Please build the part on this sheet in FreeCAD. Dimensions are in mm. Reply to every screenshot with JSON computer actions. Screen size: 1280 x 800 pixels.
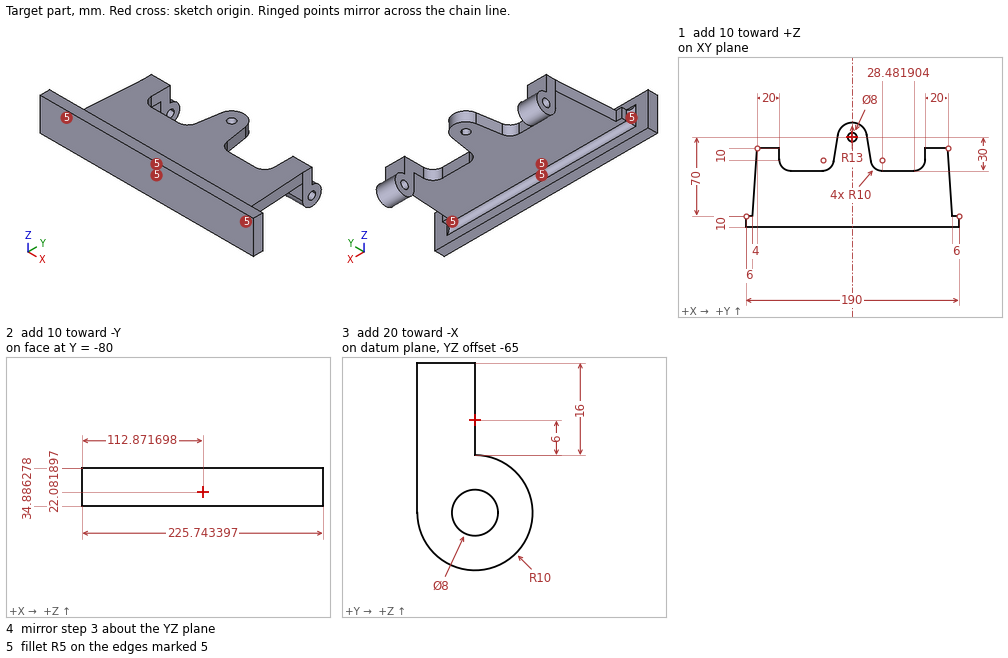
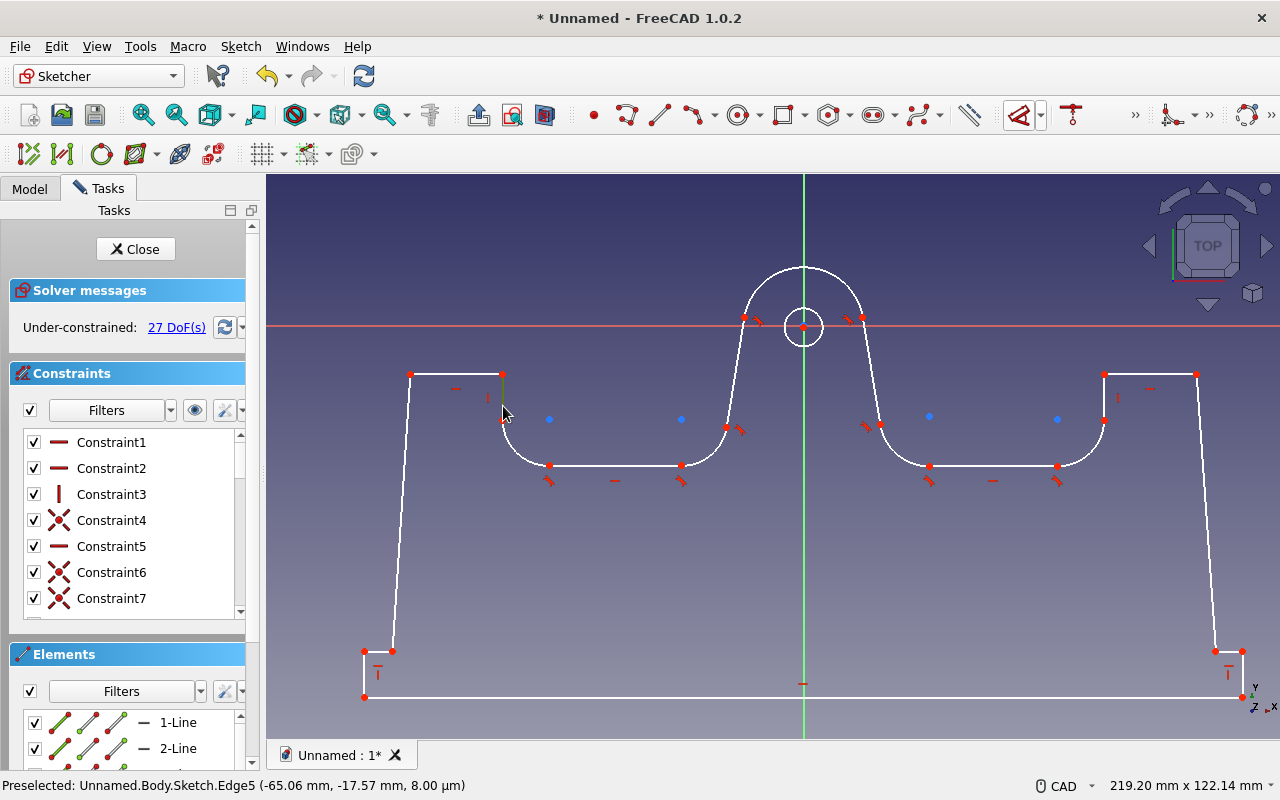
{"action": "left_click", "coordinate": [508, 441]}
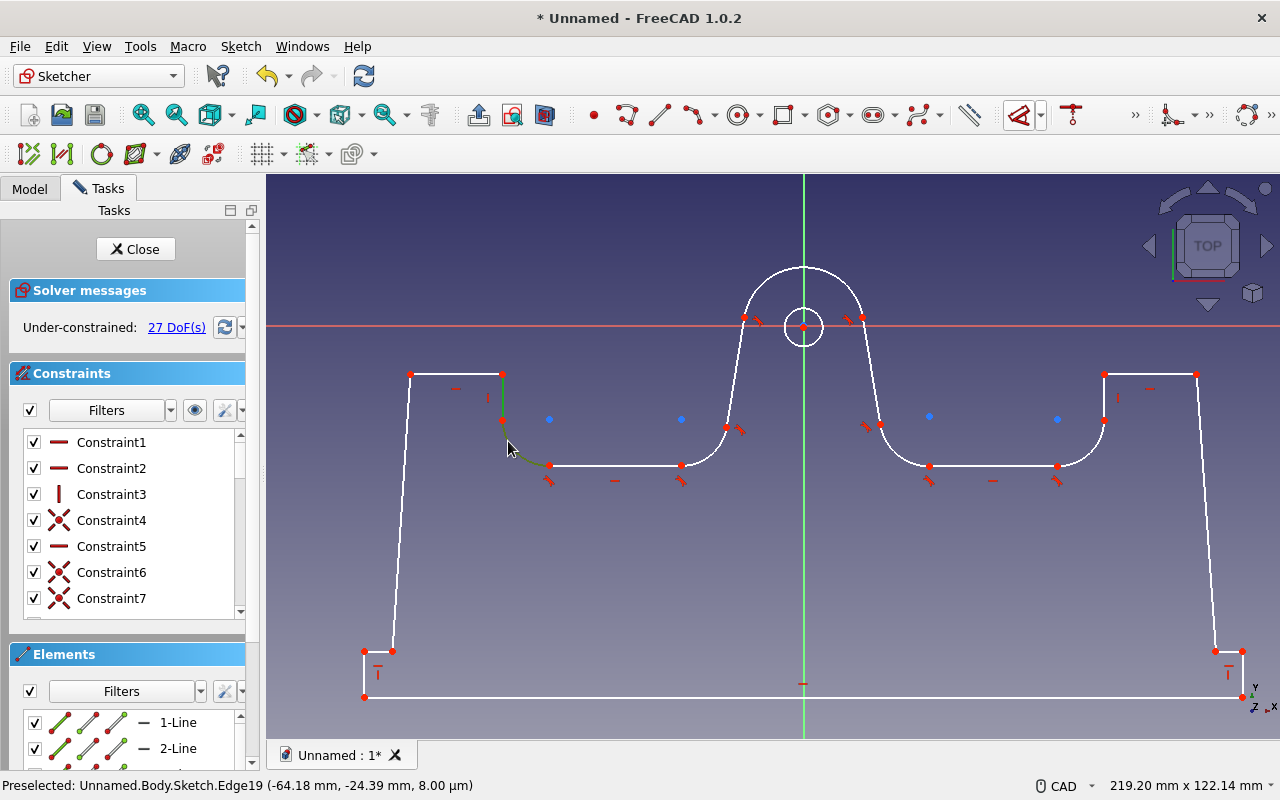
{"action": "key", "text": "t"}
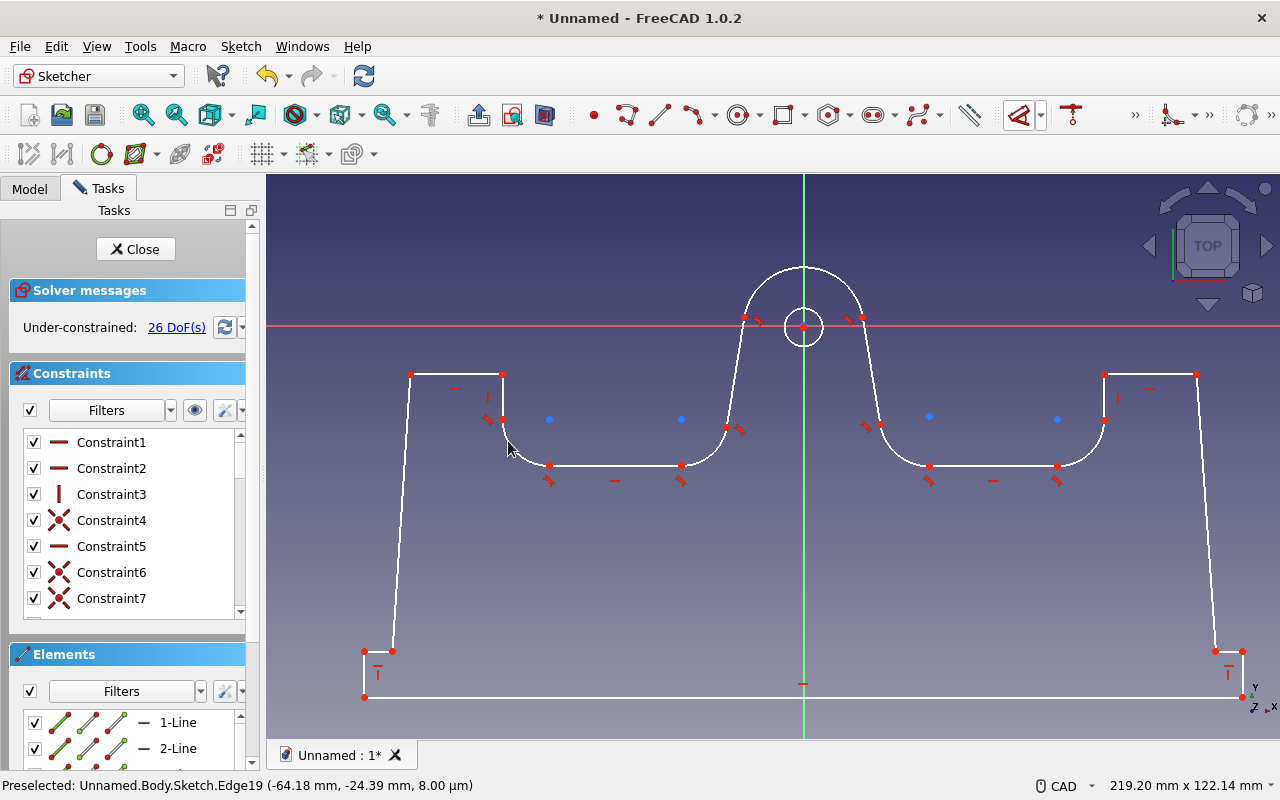
{"action": "left_click", "coordinate": [1104, 388]}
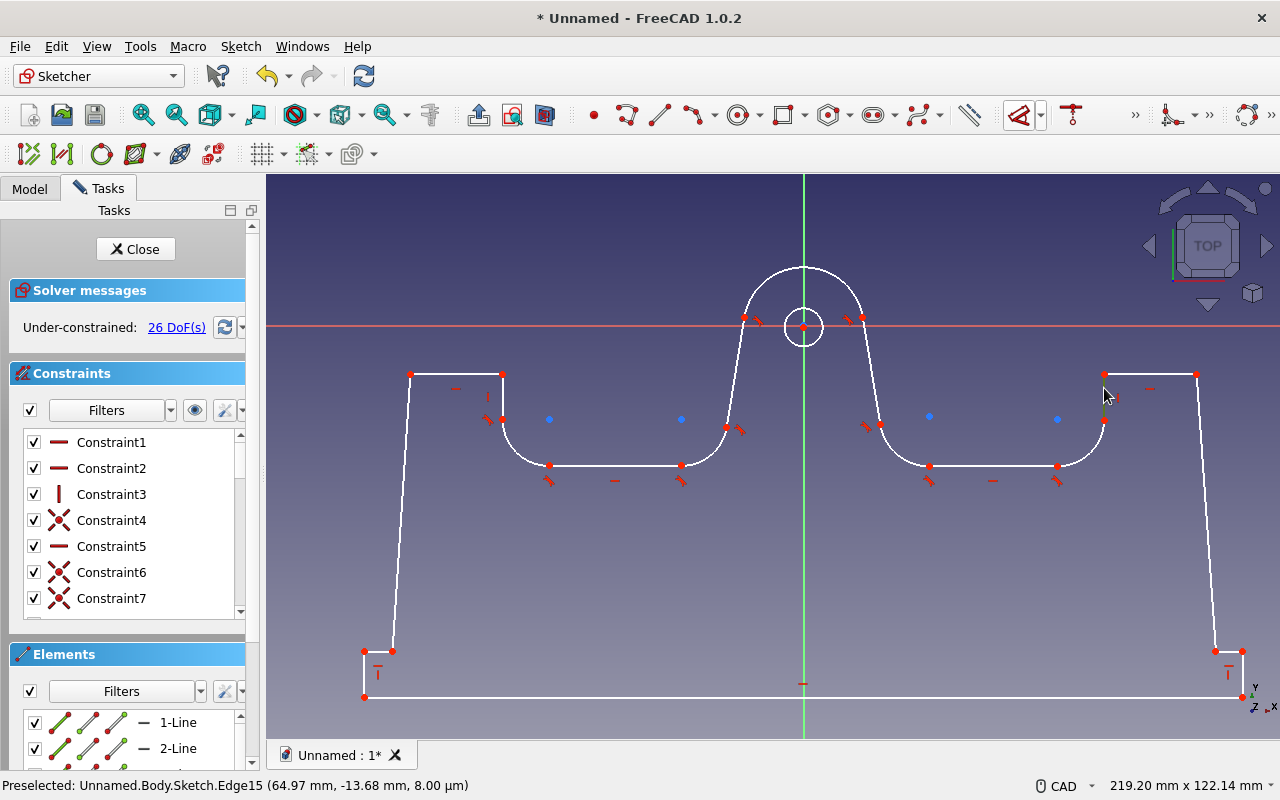
{"action": "left_click", "coordinate": [1078, 461]}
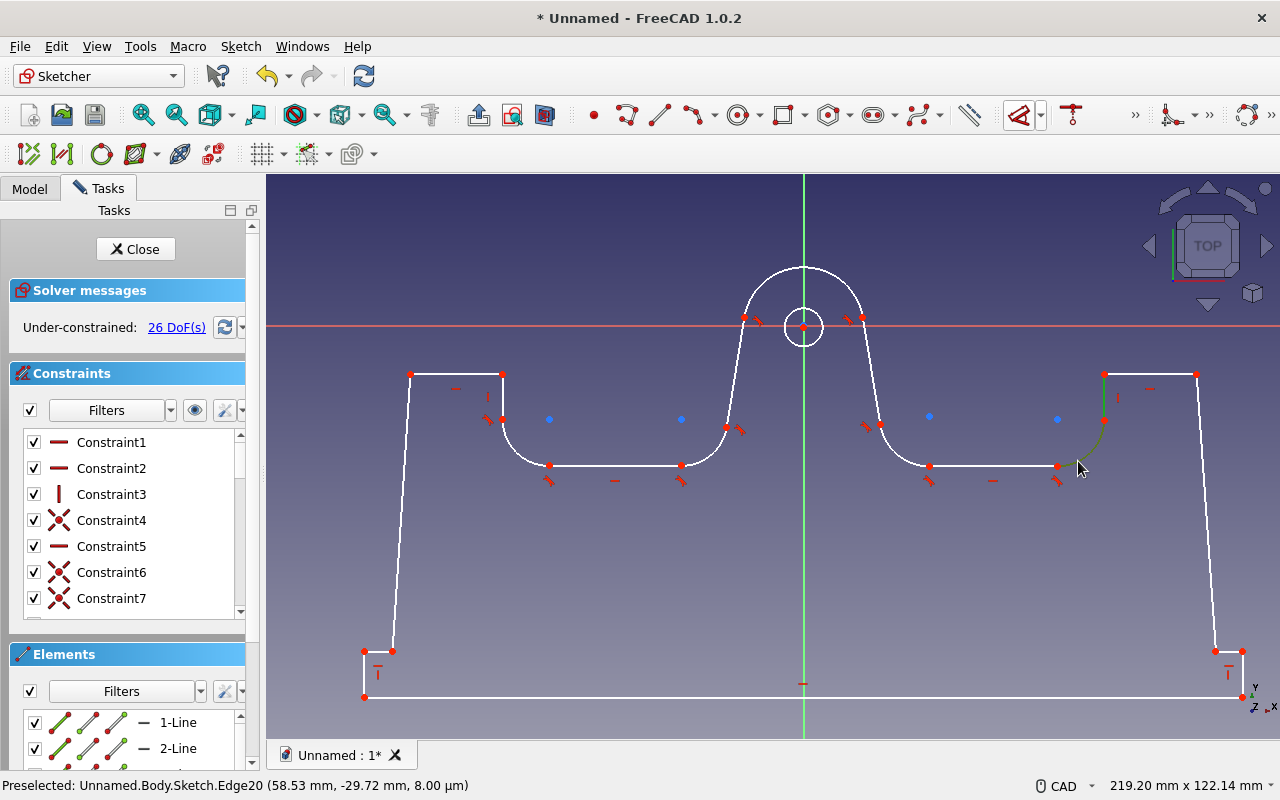
{"action": "key", "text": "t"}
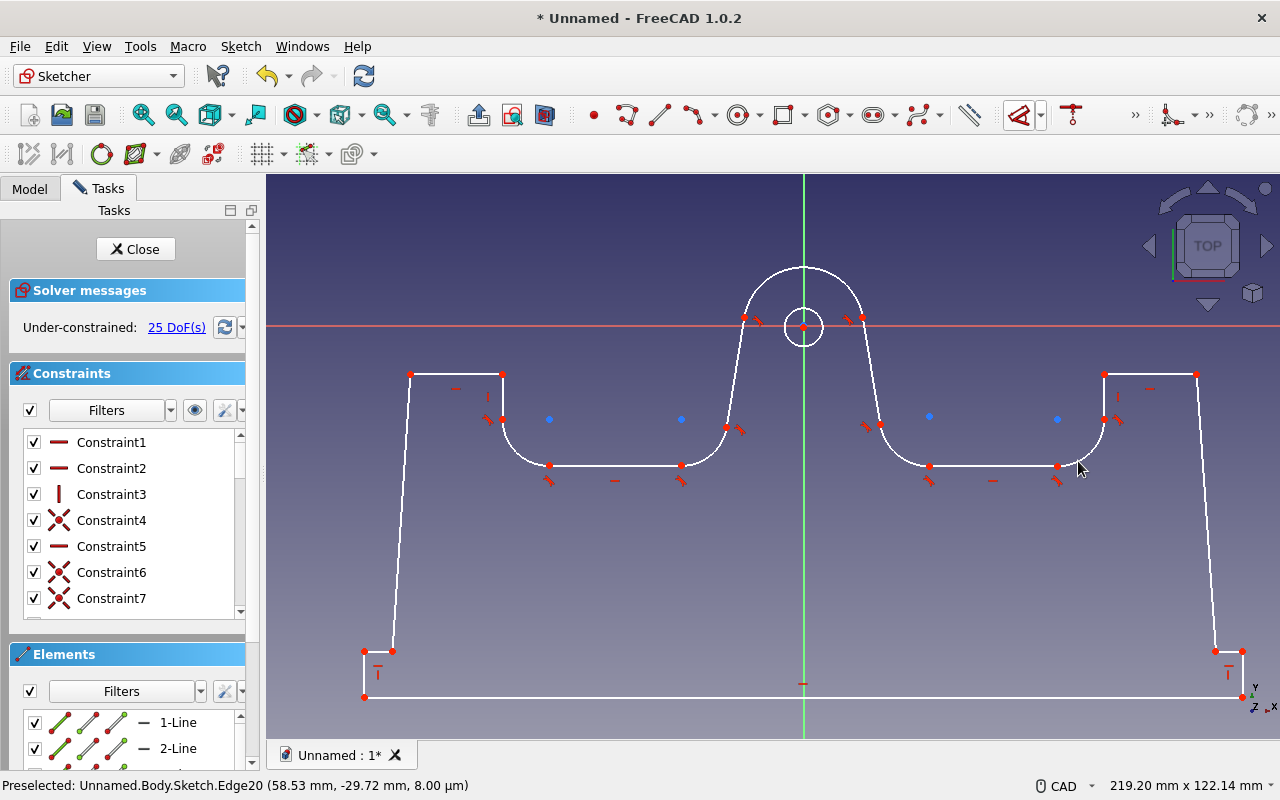
{"action": "scroll", "coordinate": [804, 327], "scroll_direction": "up", "scroll_amount": 4}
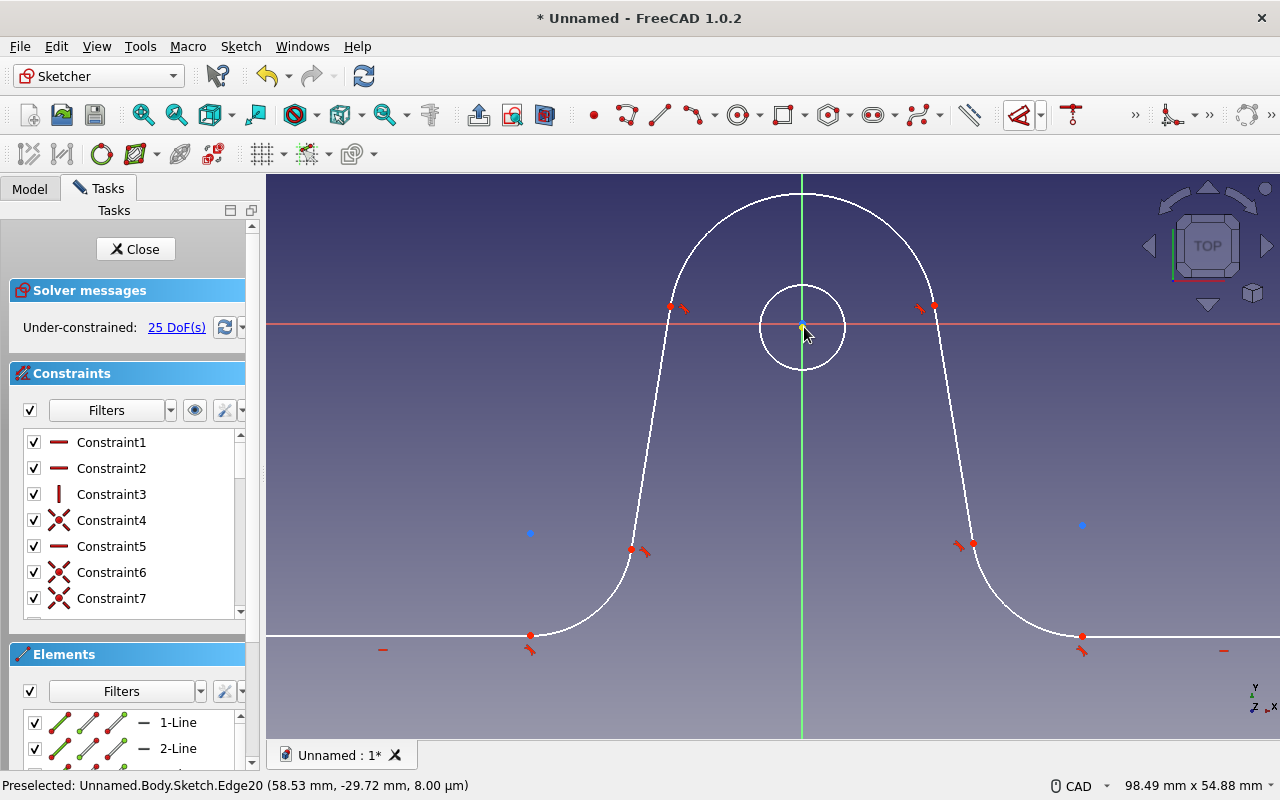
{"action": "left_click_drag", "start_coordinate": [792, 314], "coordinate": [812, 337]}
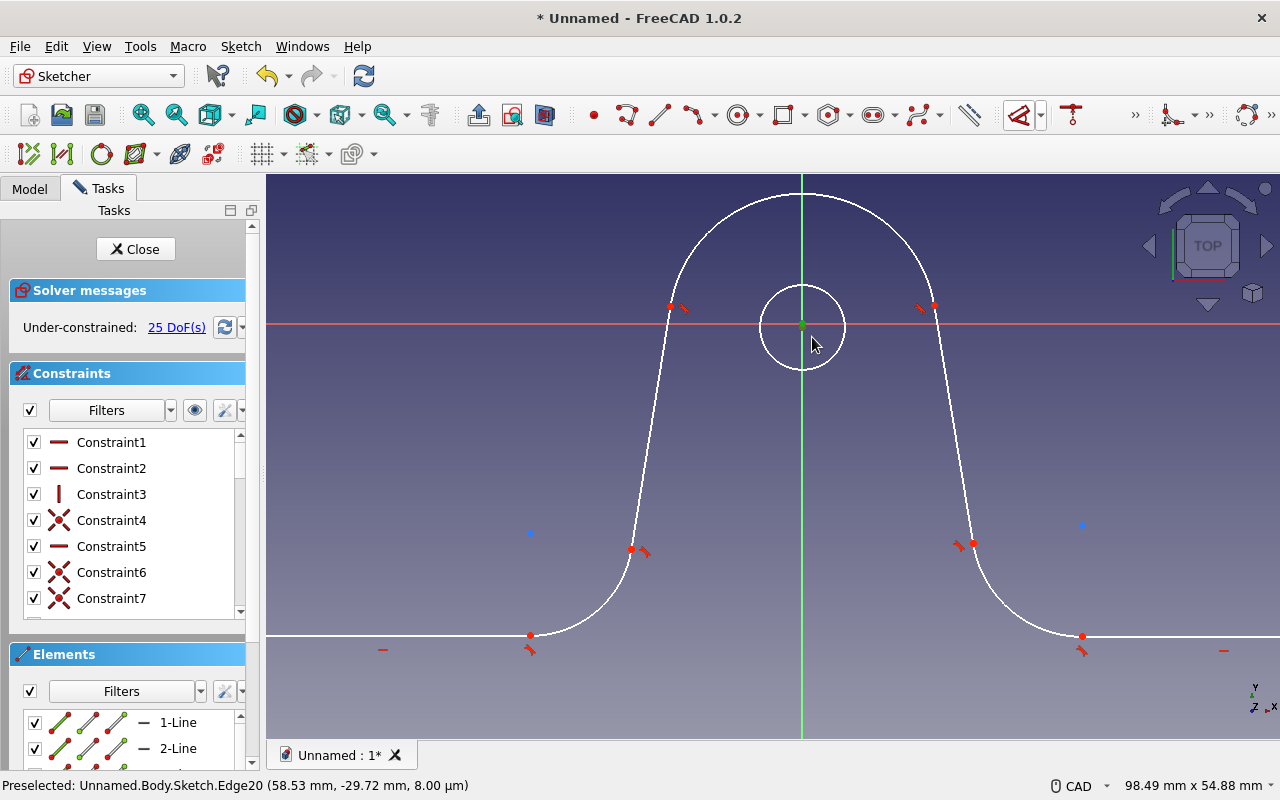
{"action": "key", "text": "c"}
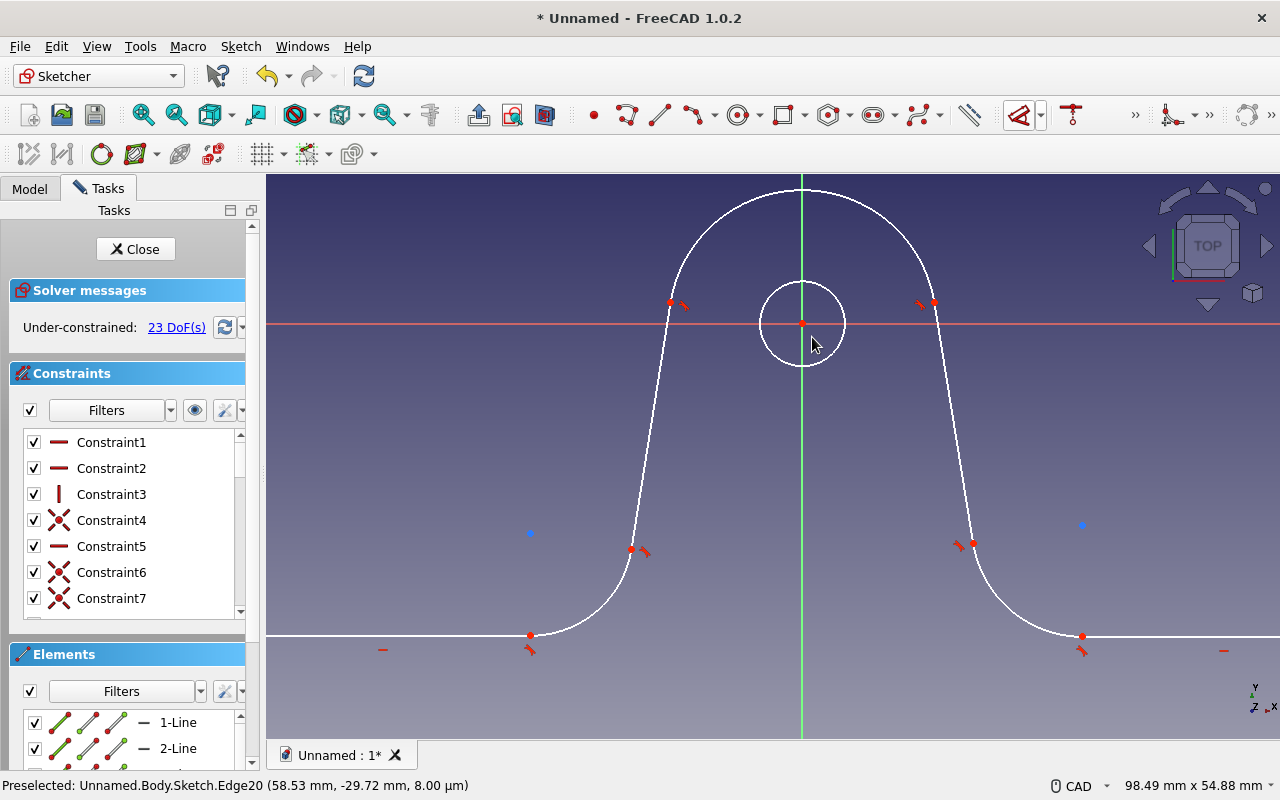
{"action": "left_click", "coordinate": [990, 587]}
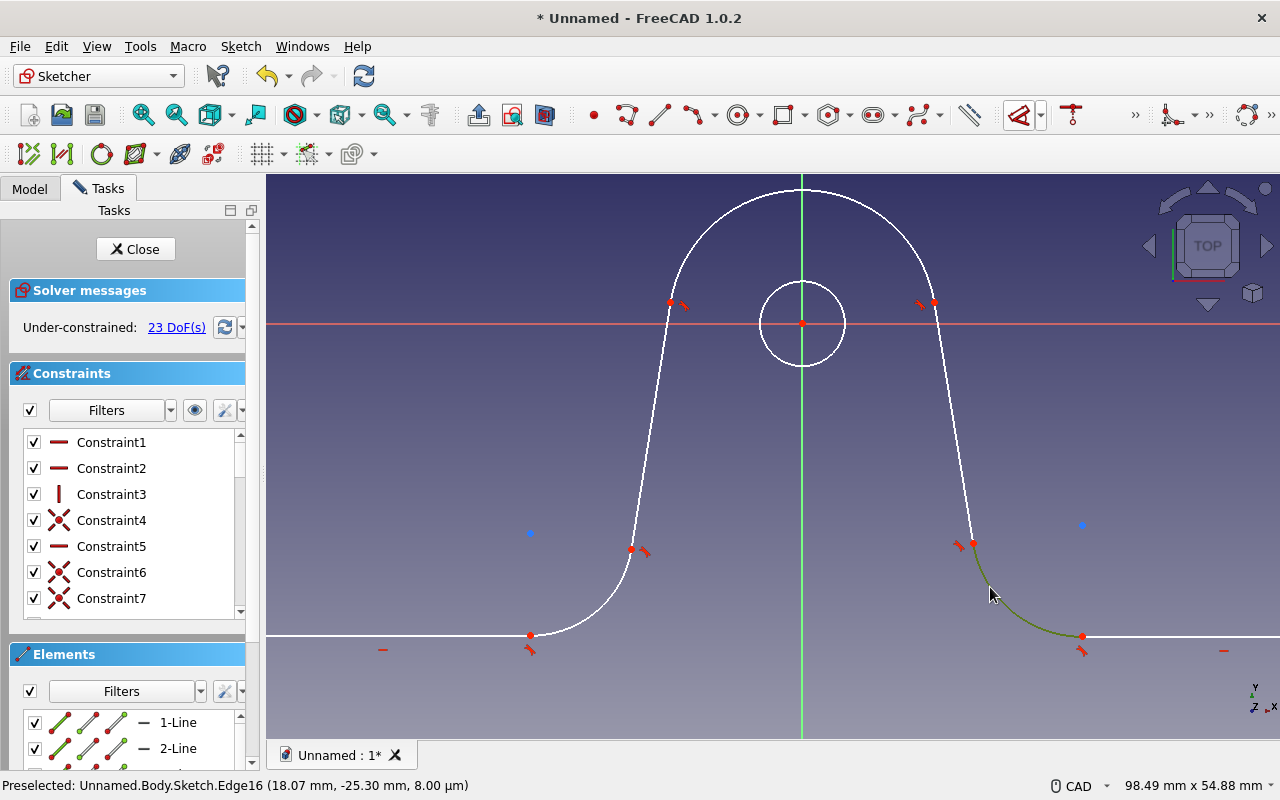
{"action": "left_click", "coordinate": [572, 627]}